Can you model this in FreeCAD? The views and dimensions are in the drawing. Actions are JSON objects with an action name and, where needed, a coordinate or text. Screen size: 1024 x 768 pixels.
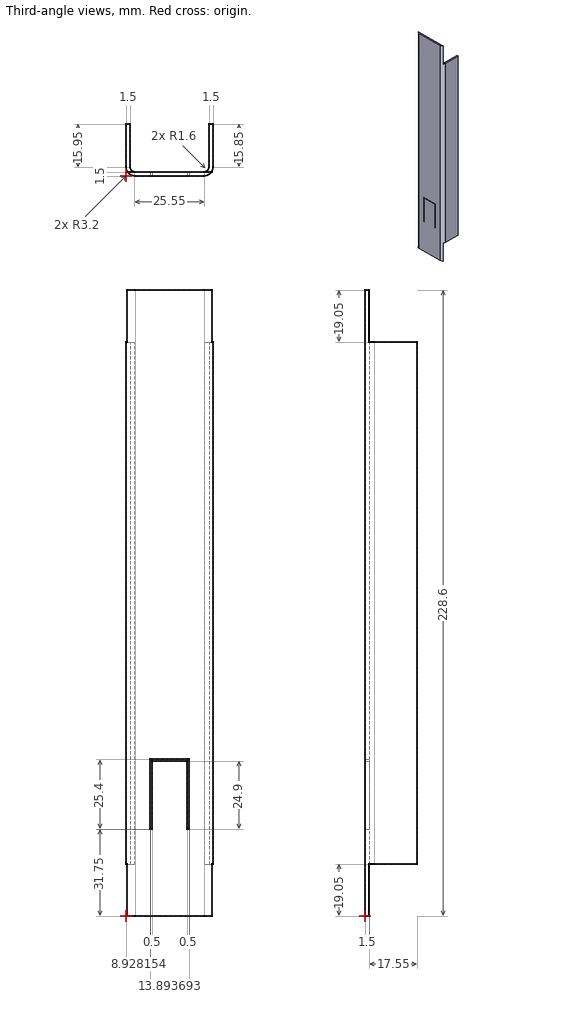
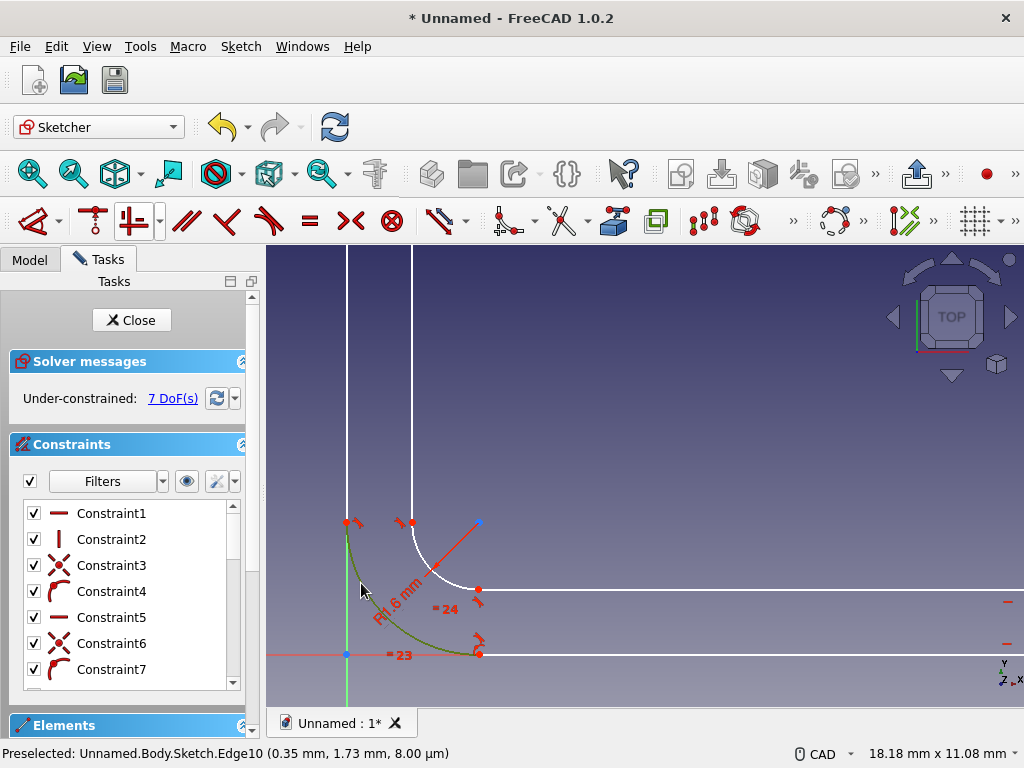
{"action": "left_click", "coordinate": [58, 222]}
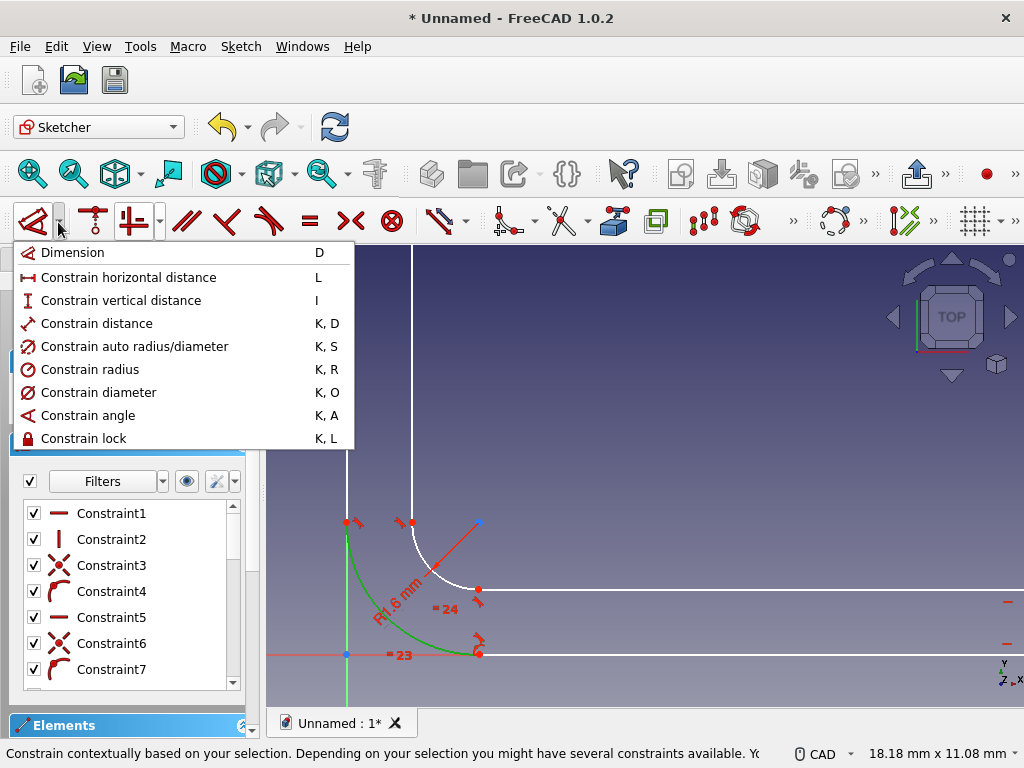
{"action": "left_click", "coordinate": [184, 370]}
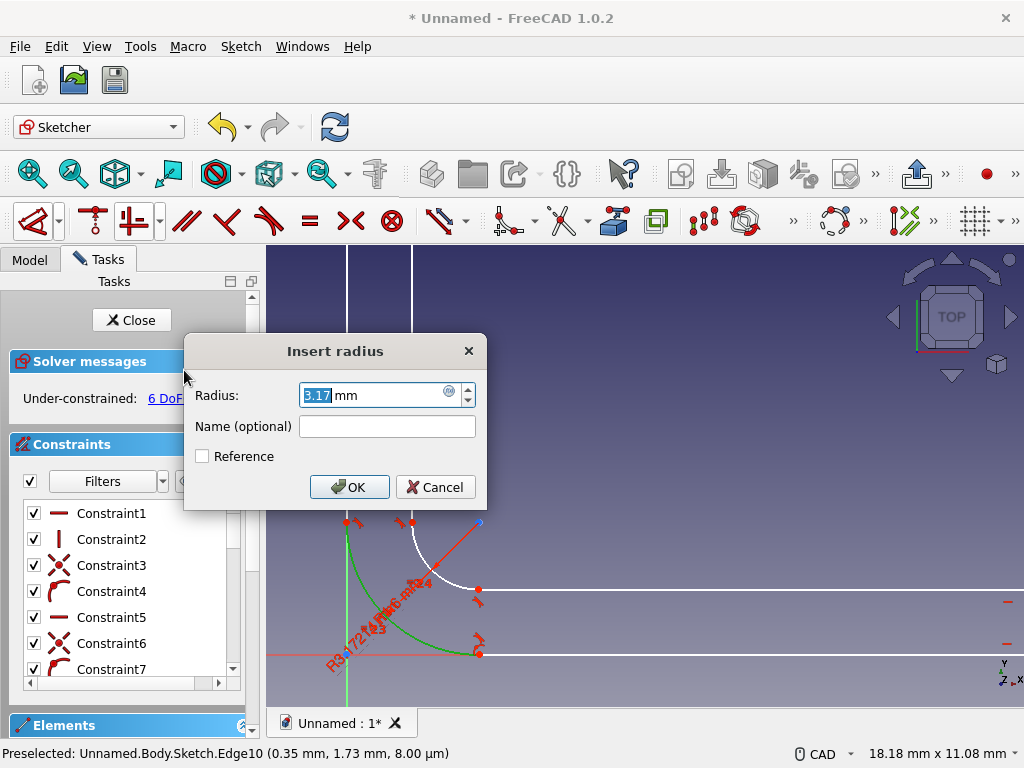
{"action": "type", "text": "3.2"}
{"action": "key", "text": "Return"}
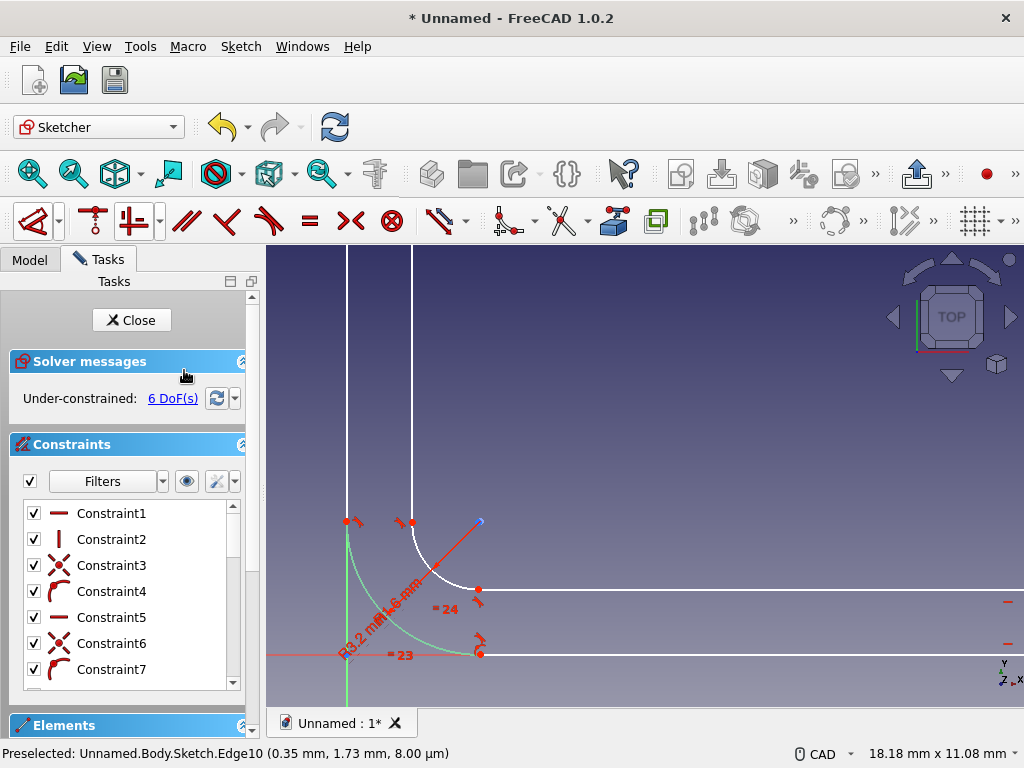
{"action": "scroll", "coordinate": [390, 570], "scroll_direction": "down", "scroll_amount": 6}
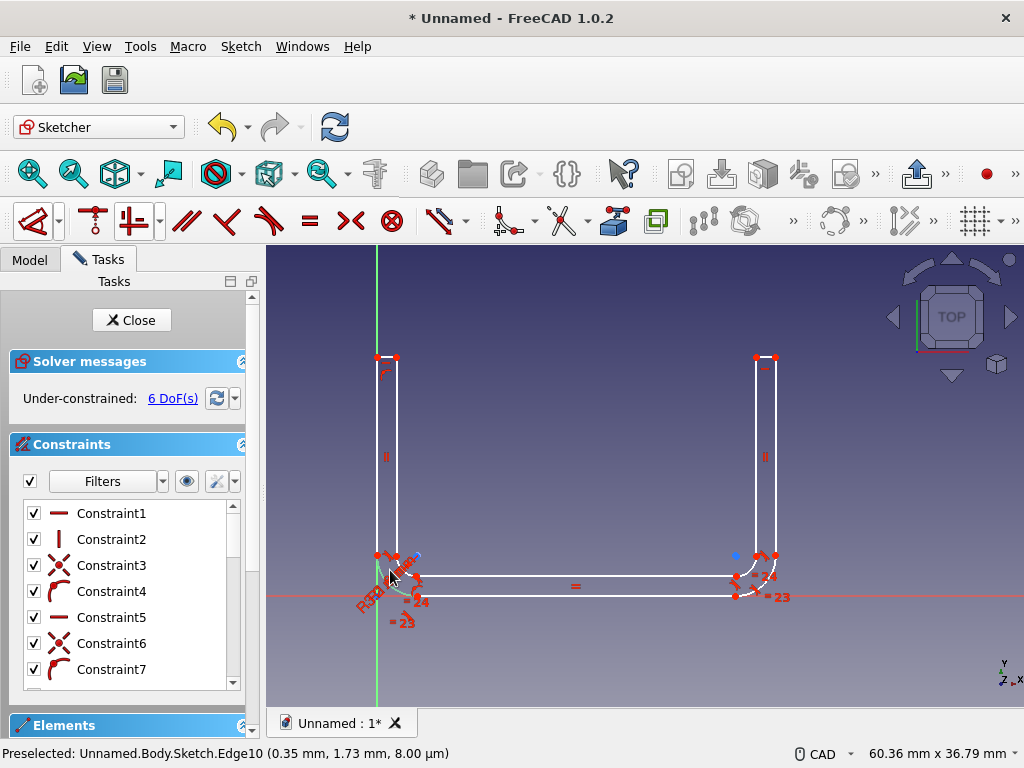
{"action": "scroll", "coordinate": [391, 357], "scroll_direction": "up", "scroll_amount": 5}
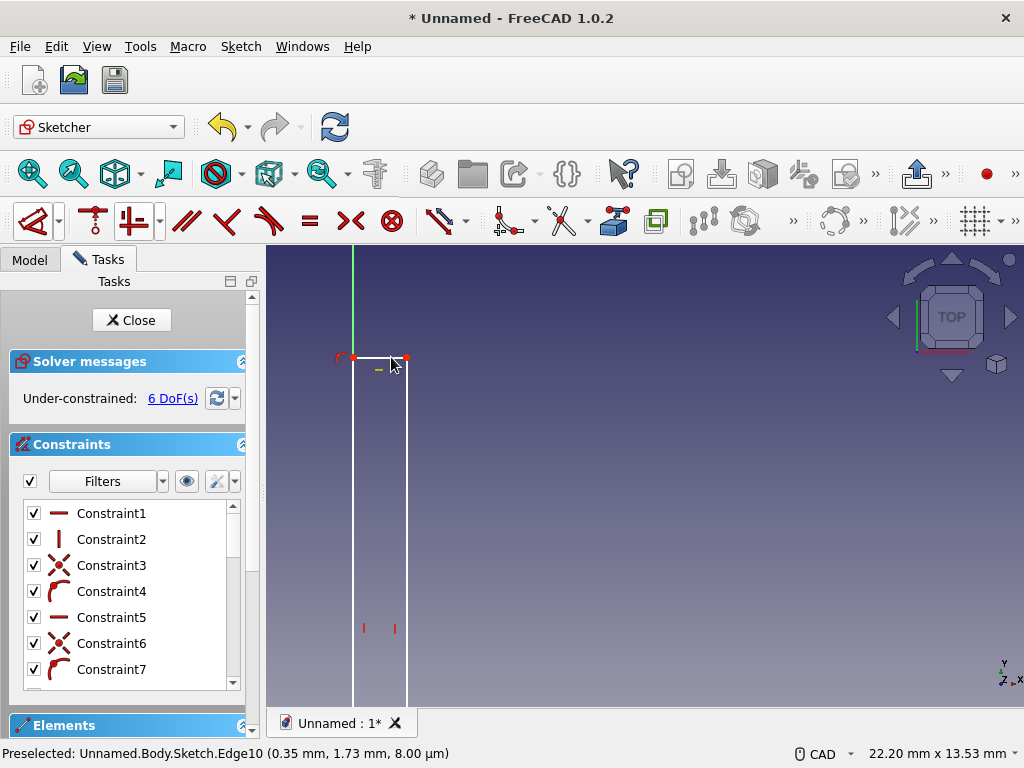
{"action": "left_click", "coordinate": [390, 358]}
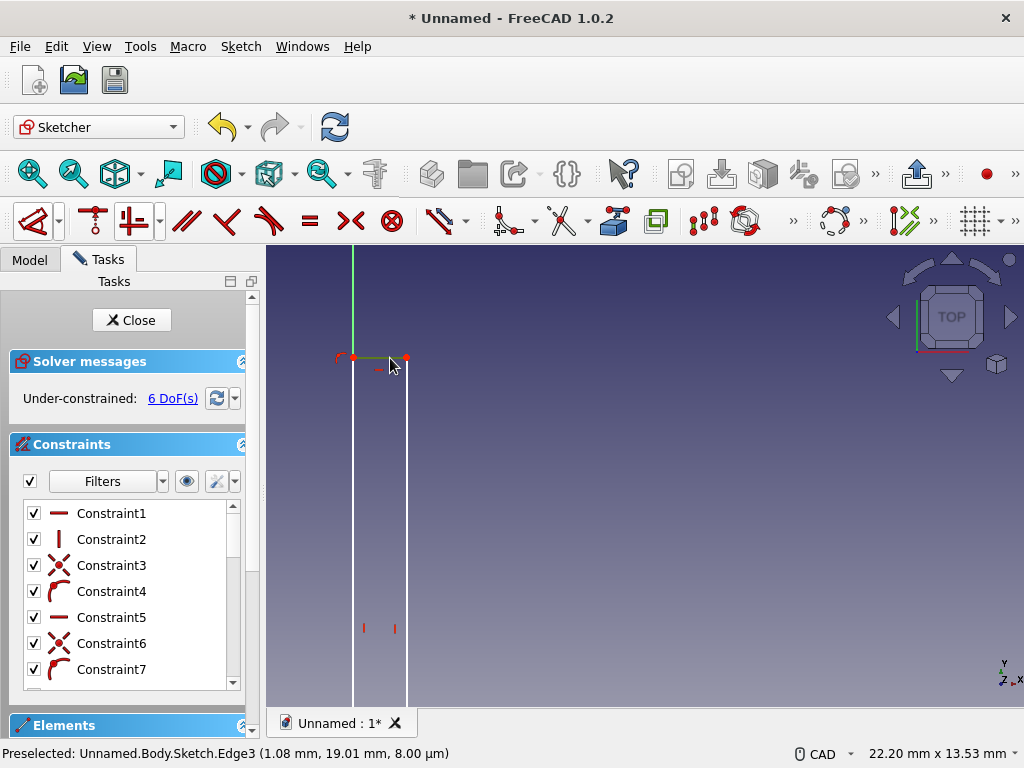
{"action": "left_click", "coordinate": [58, 222]}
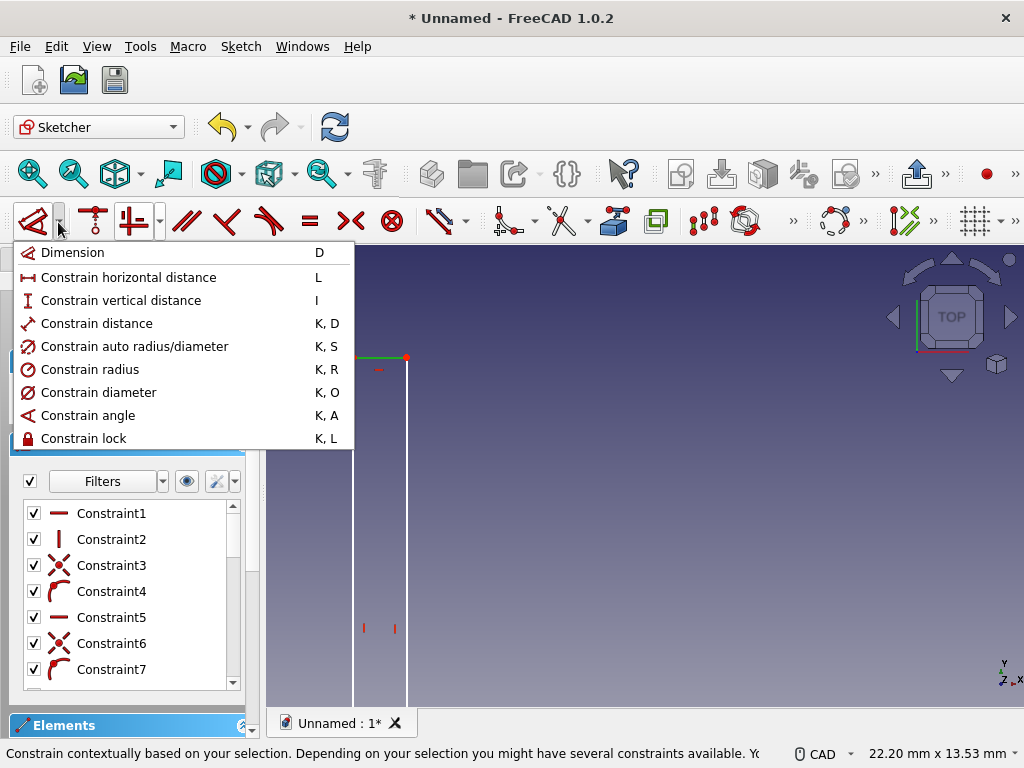
{"action": "left_click", "coordinate": [184, 278]}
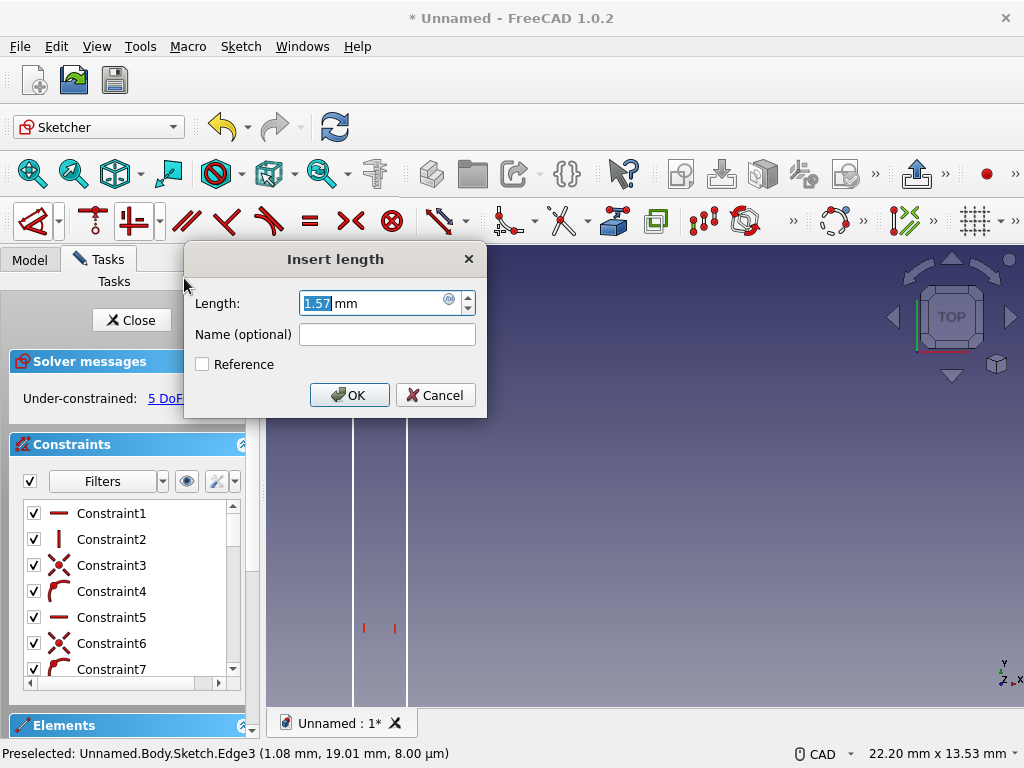
{"action": "type", "text": "1.5"}
{"action": "key", "text": "Return"}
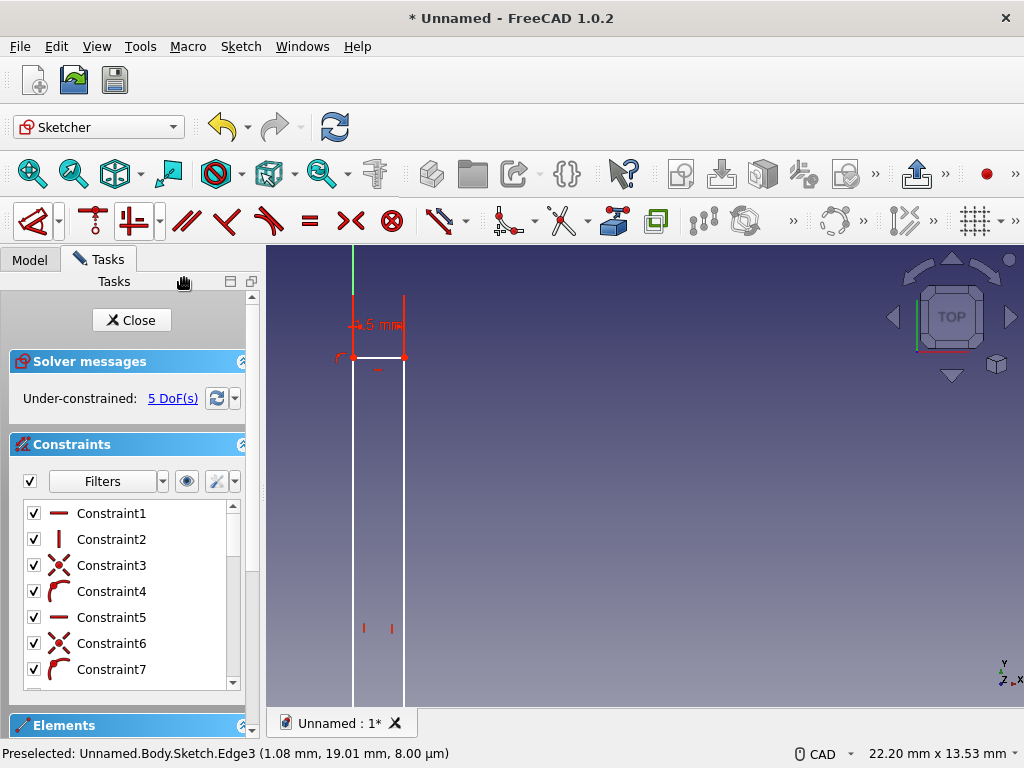
{"action": "scroll", "coordinate": [391, 357], "scroll_direction": "down", "scroll_amount": 5}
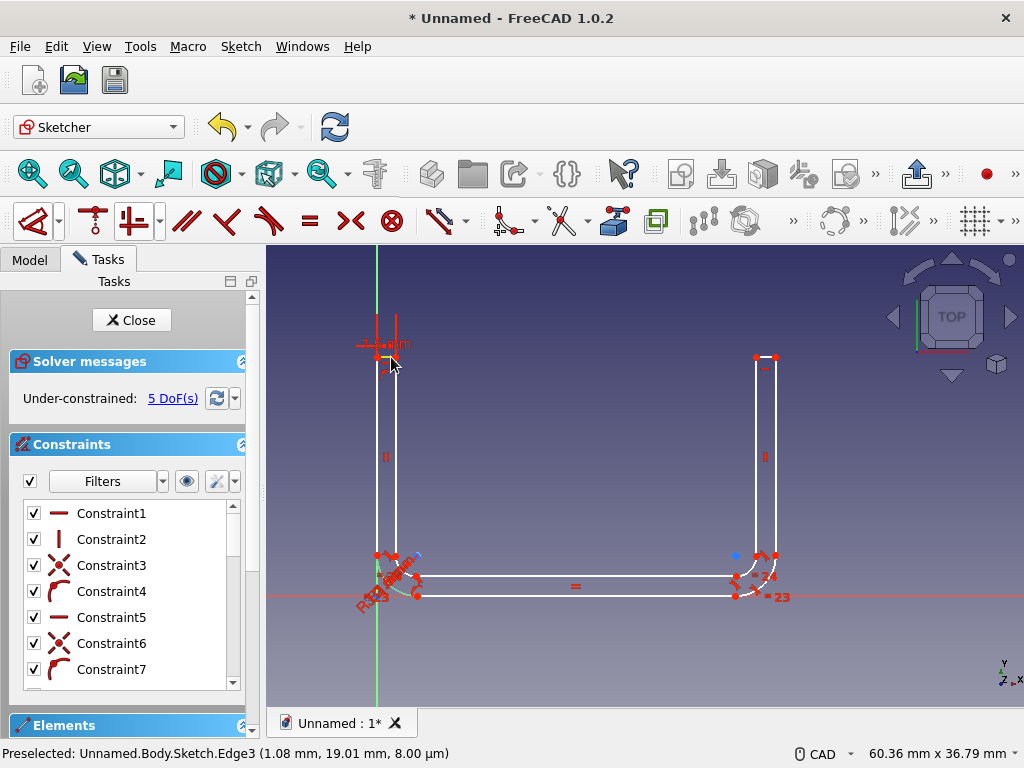
{"action": "scroll", "coordinate": [770, 357], "scroll_direction": "up", "scroll_amount": 5}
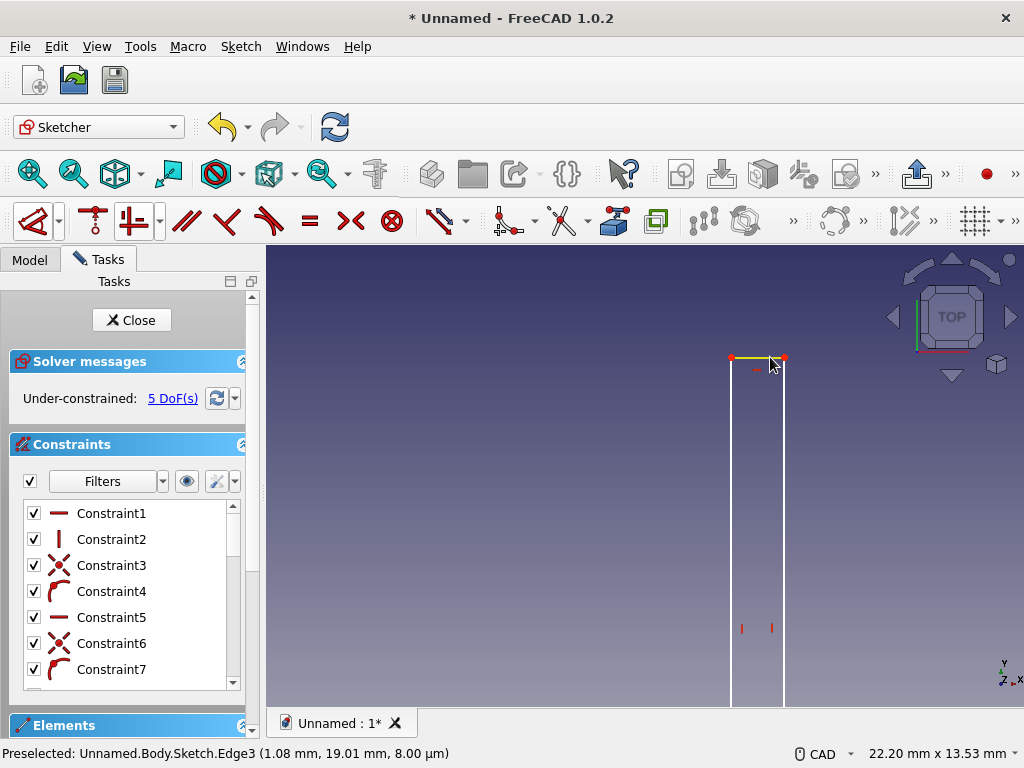
{"action": "left_click", "coordinate": [768, 358]}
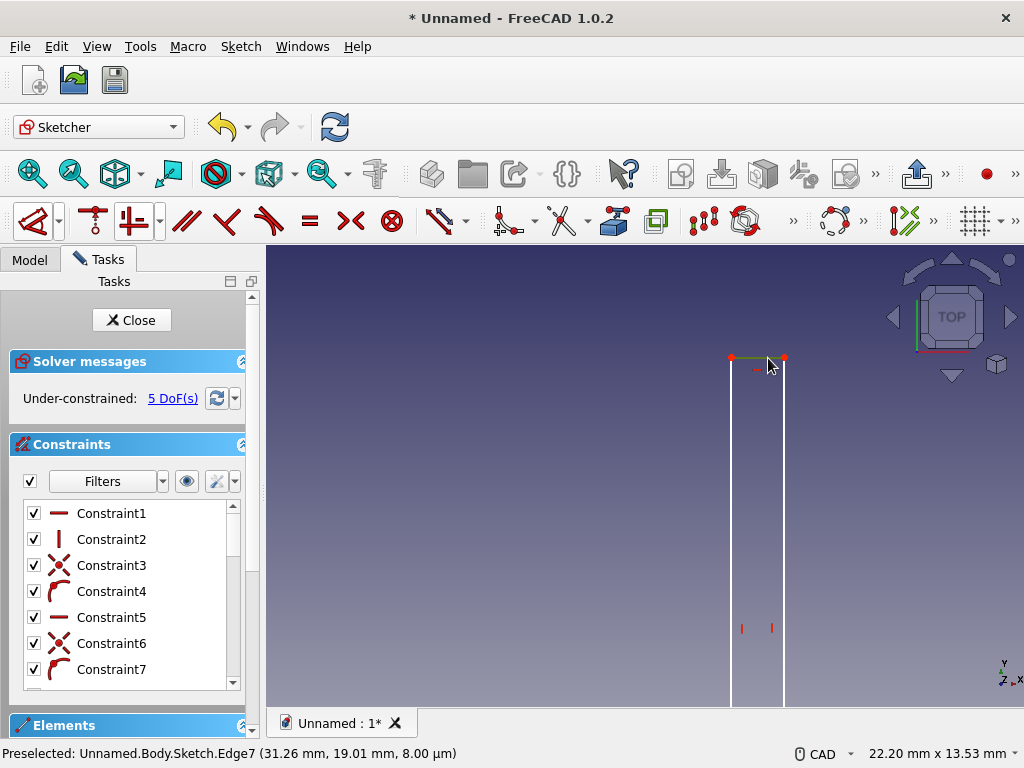
{"action": "key", "text": "l"}